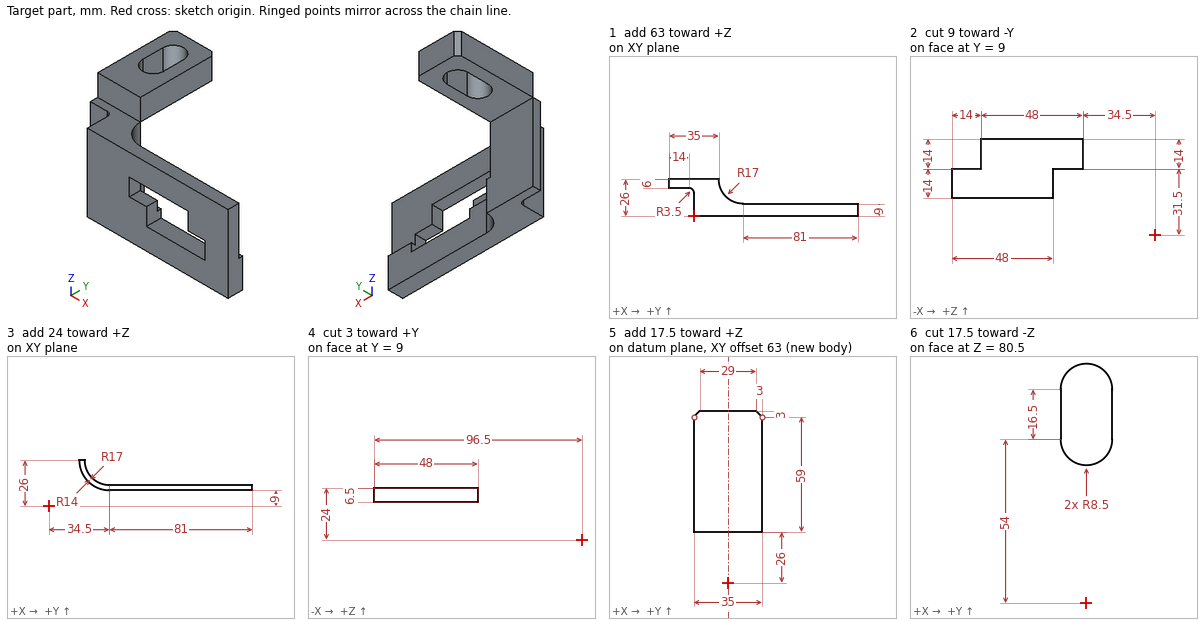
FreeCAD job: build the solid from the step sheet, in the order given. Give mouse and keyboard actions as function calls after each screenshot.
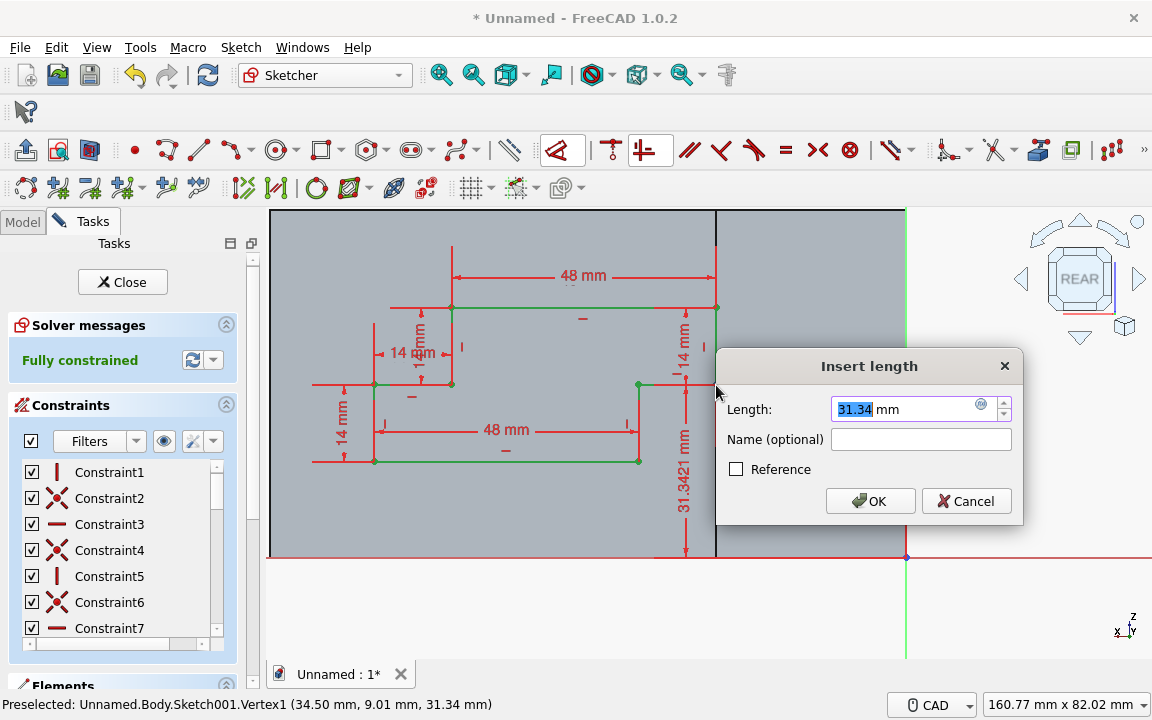
text(31.5)
key(Return)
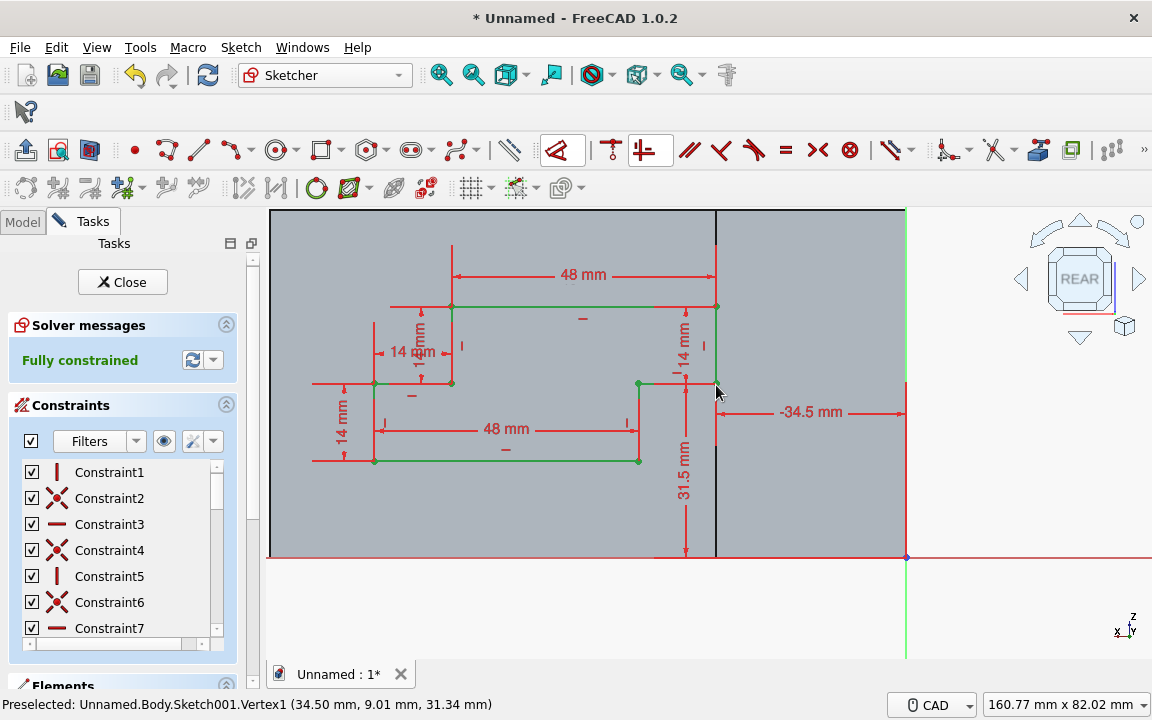
click(123, 282)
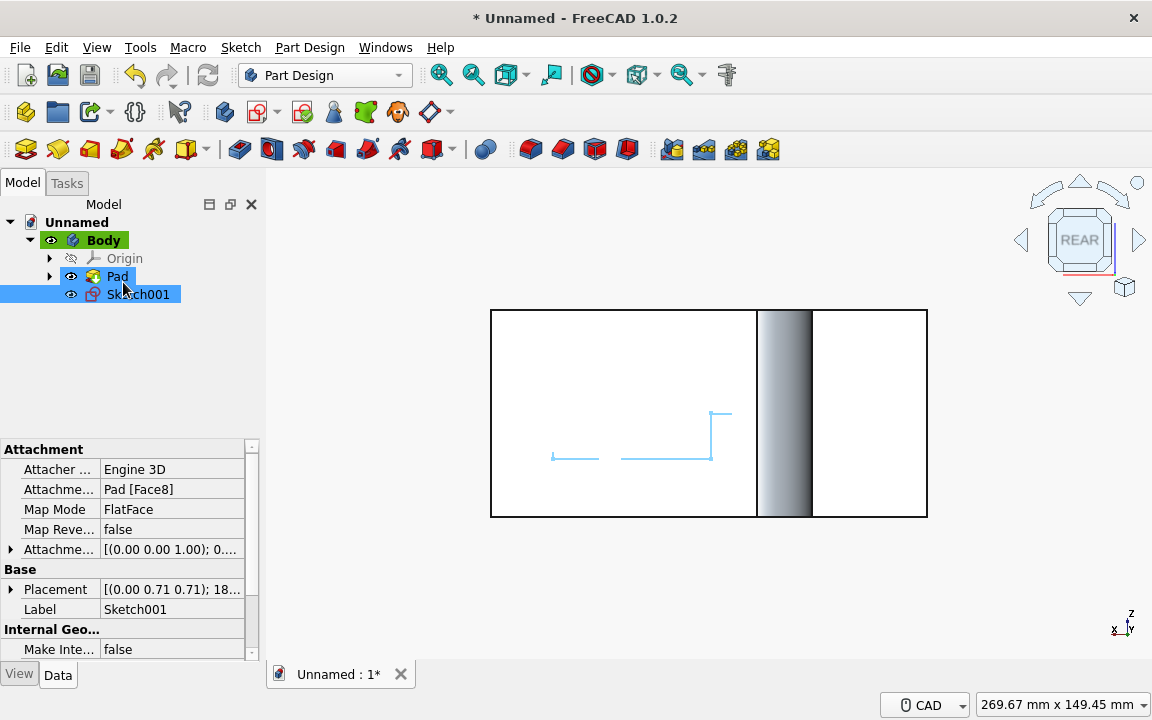
click(240, 150)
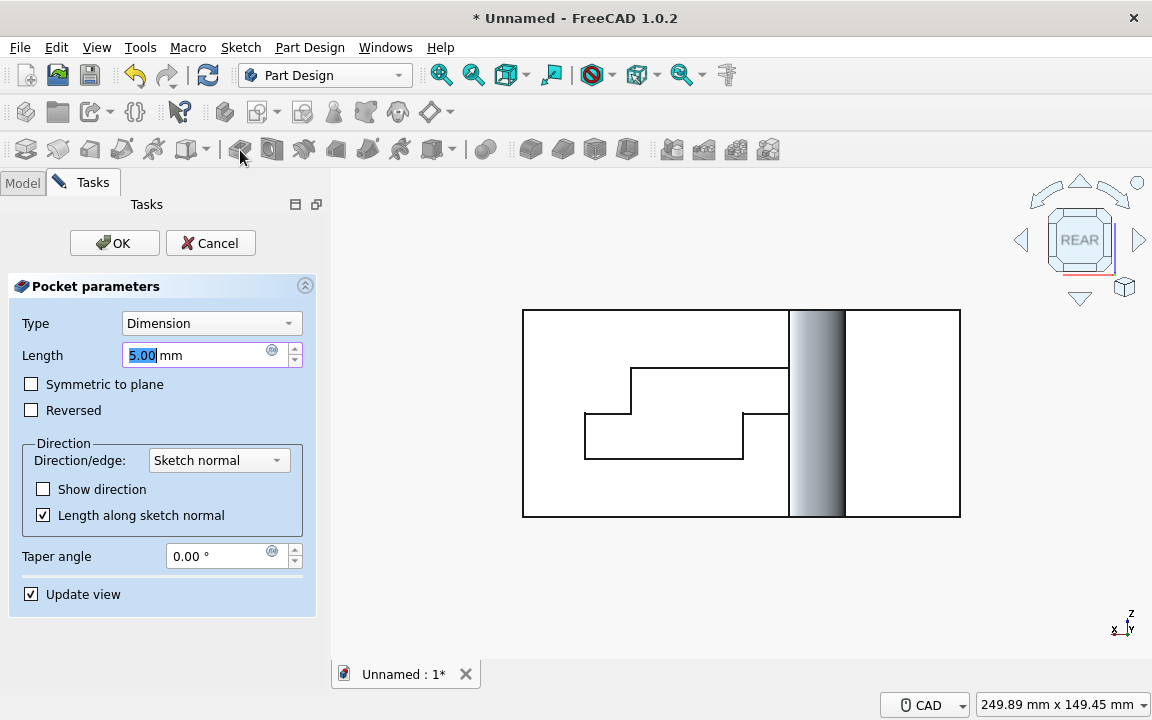
text(9)
key(Tab)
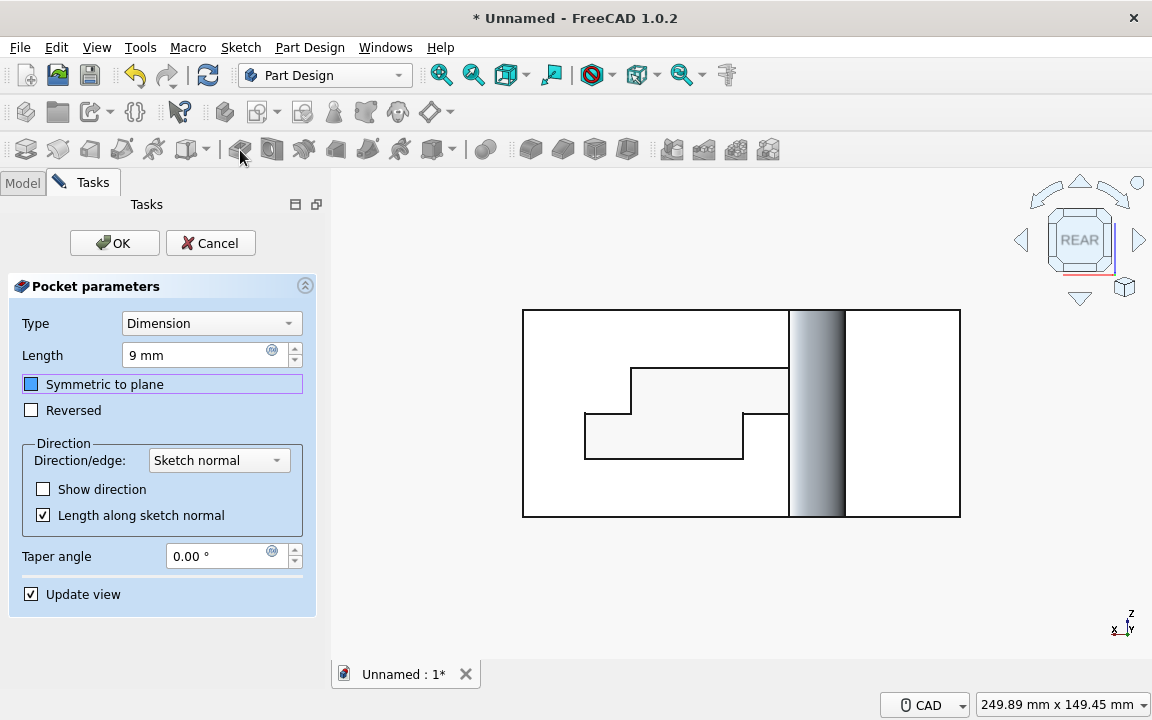
click(115, 243)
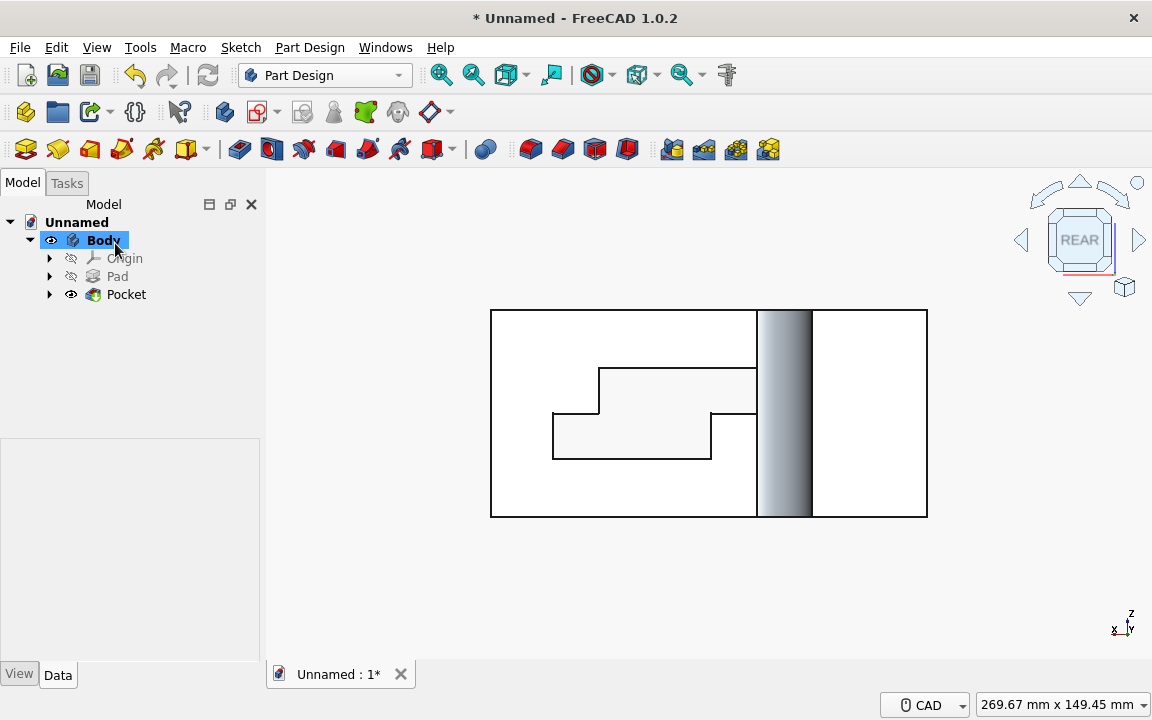
click(258, 112)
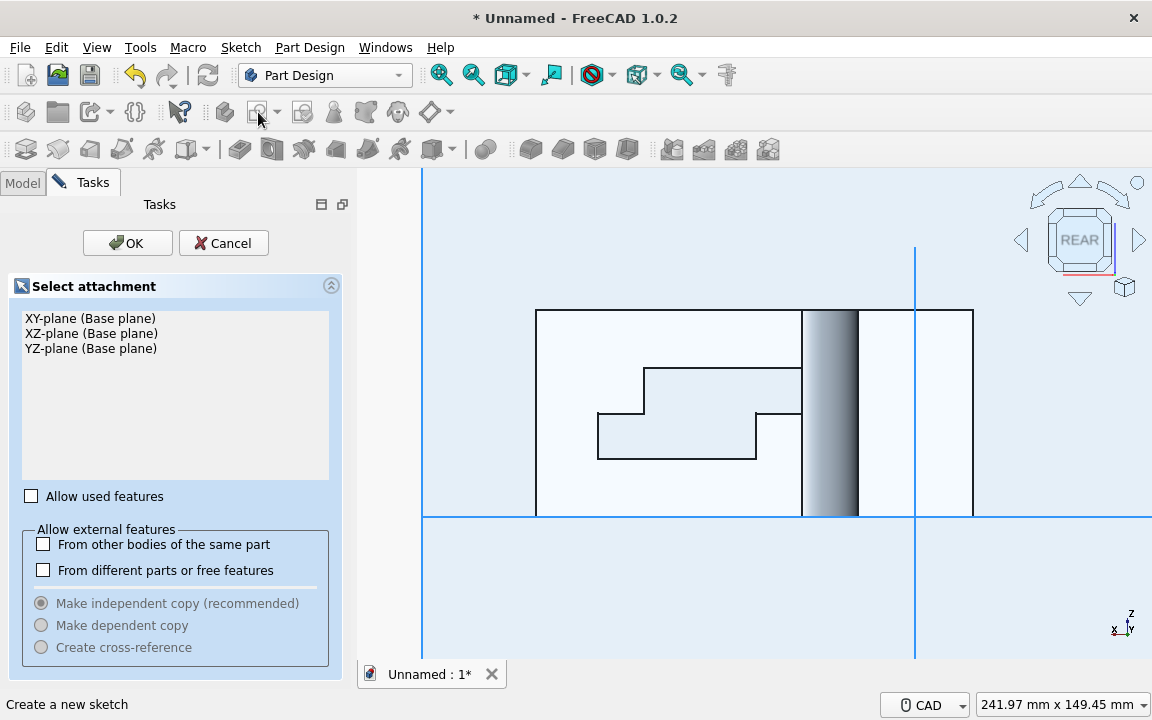
click(82, 318)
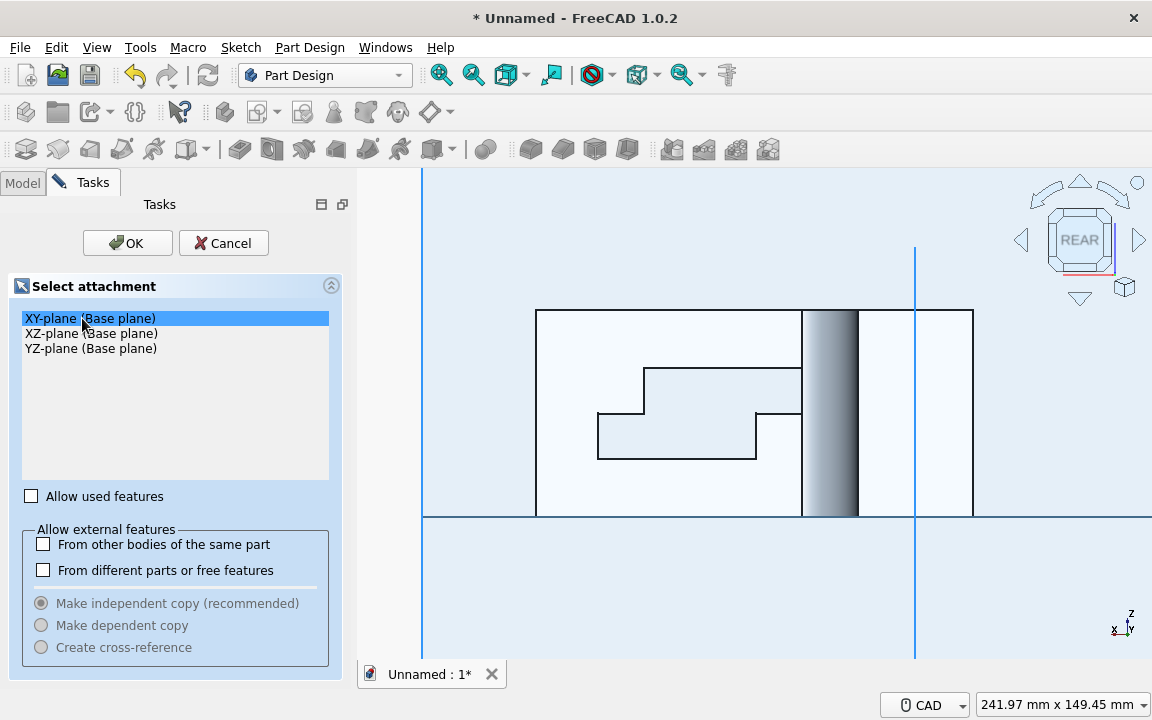
click(128, 243)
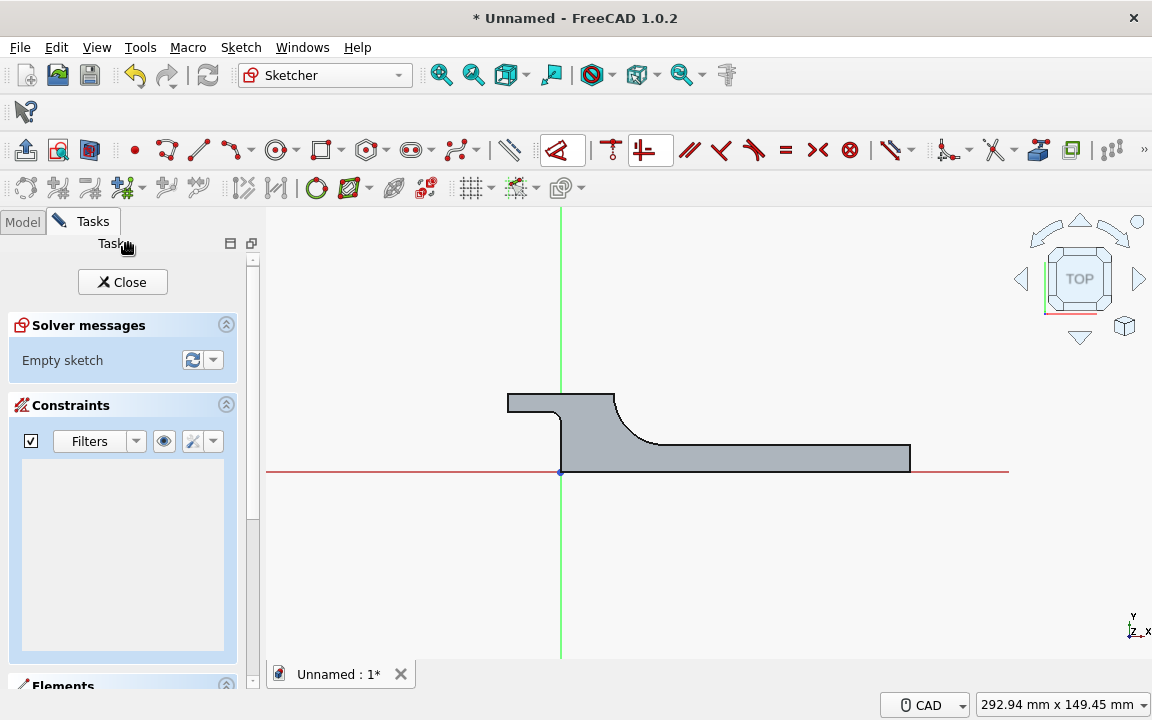
click(90, 150)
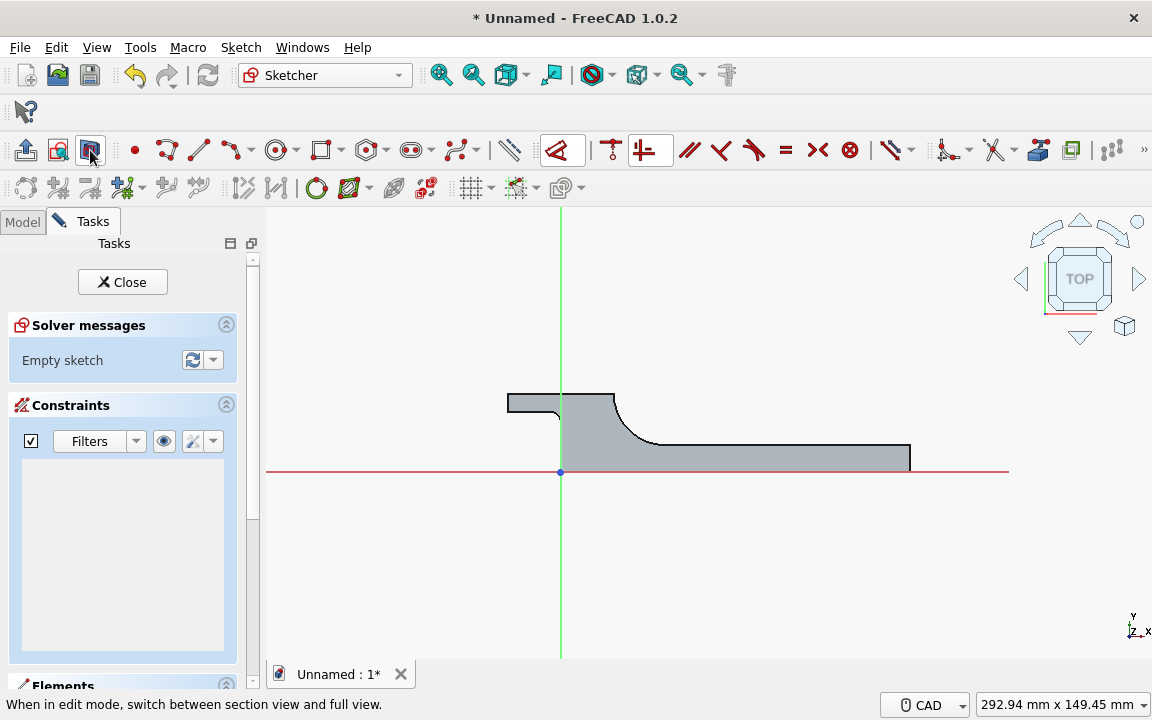
scroll(929, 433, up, 2)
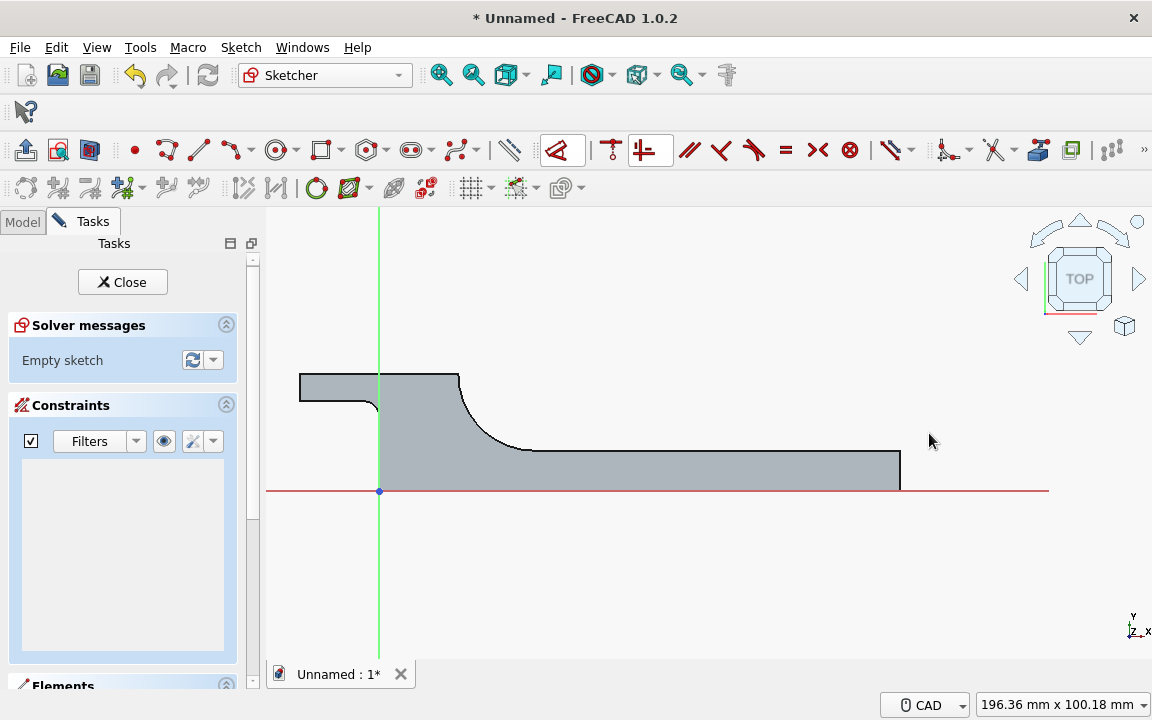
click(168, 150)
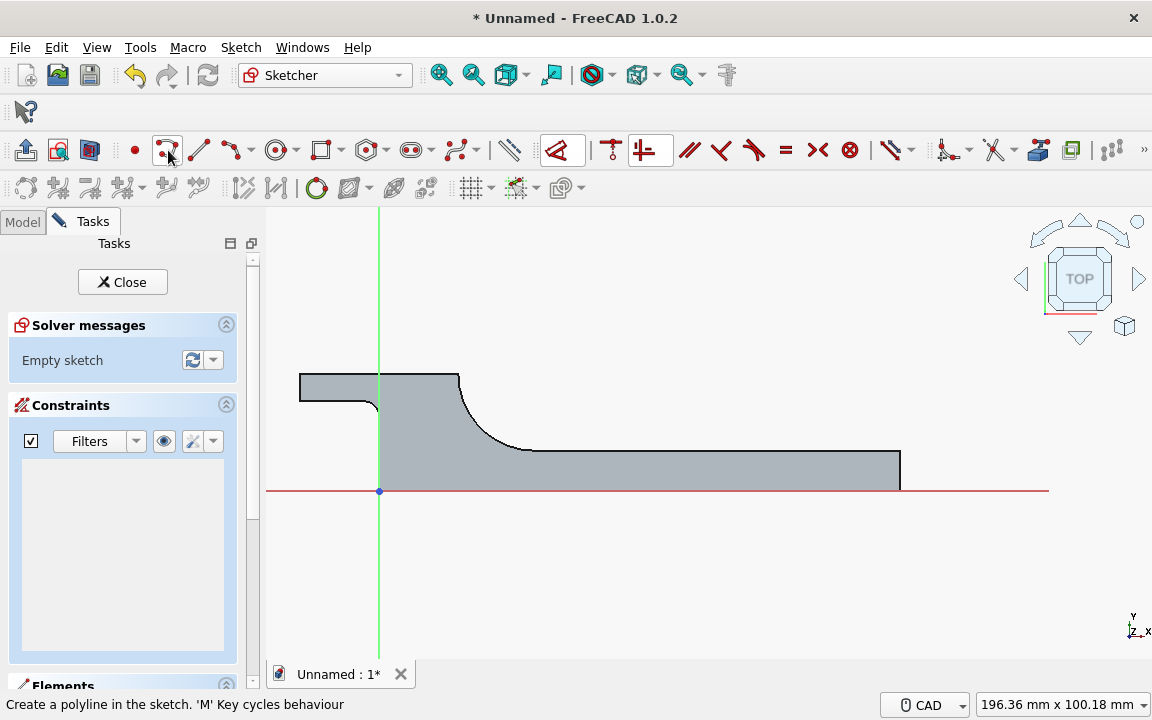
click(535, 437)
click(900, 437)
click(900, 451)
click(535, 451)
right_click(535, 451)